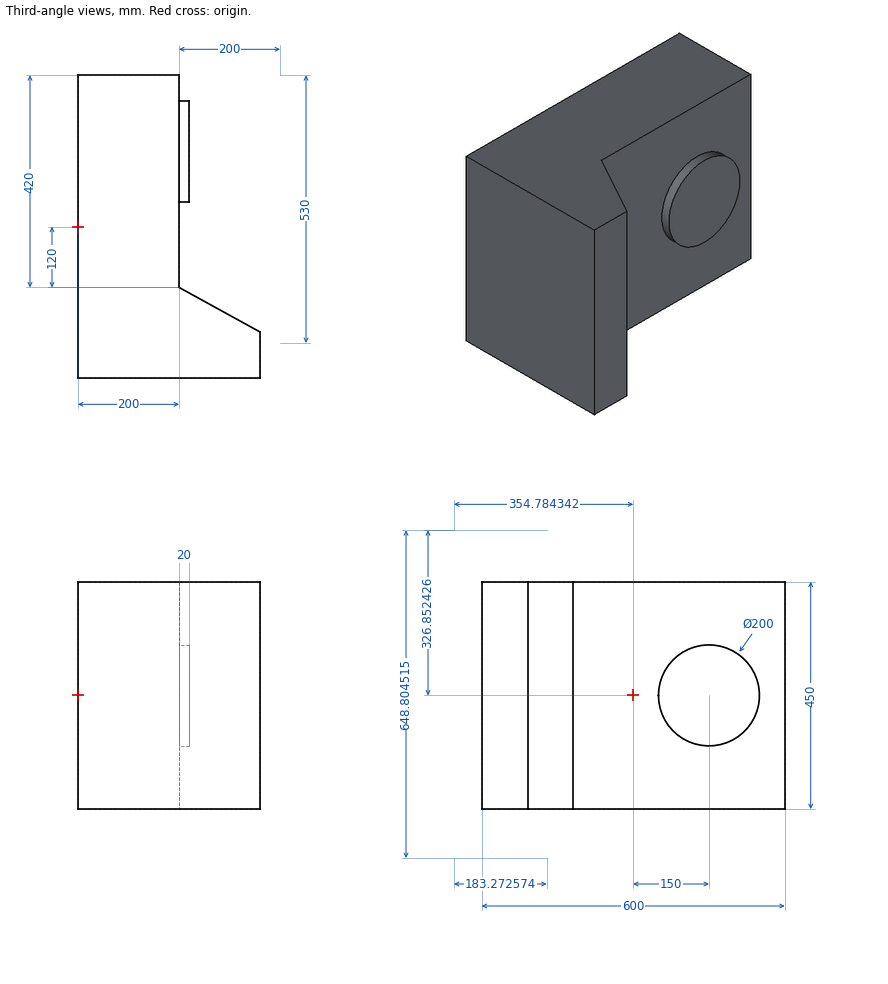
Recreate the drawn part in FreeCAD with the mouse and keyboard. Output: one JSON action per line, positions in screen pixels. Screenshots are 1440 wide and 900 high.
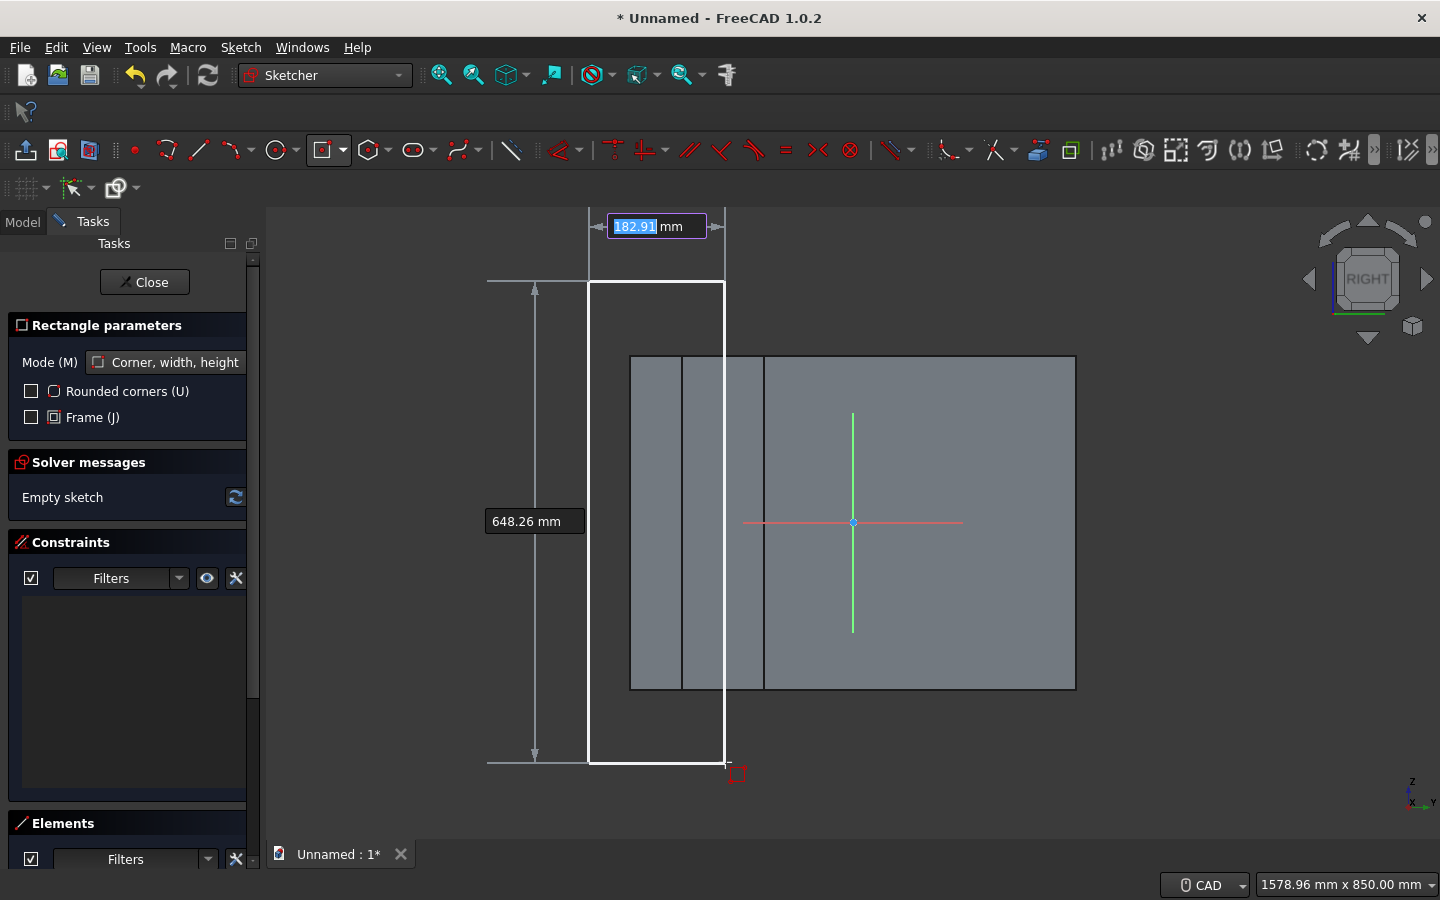
{"action": "type", "text": "183.272574"}
{"action": "key", "text": "Tab"}
{"action": "type", "text": "648.804515"}
{"action": "key", "text": "Return"}
{"action": "key", "text": "Escape"}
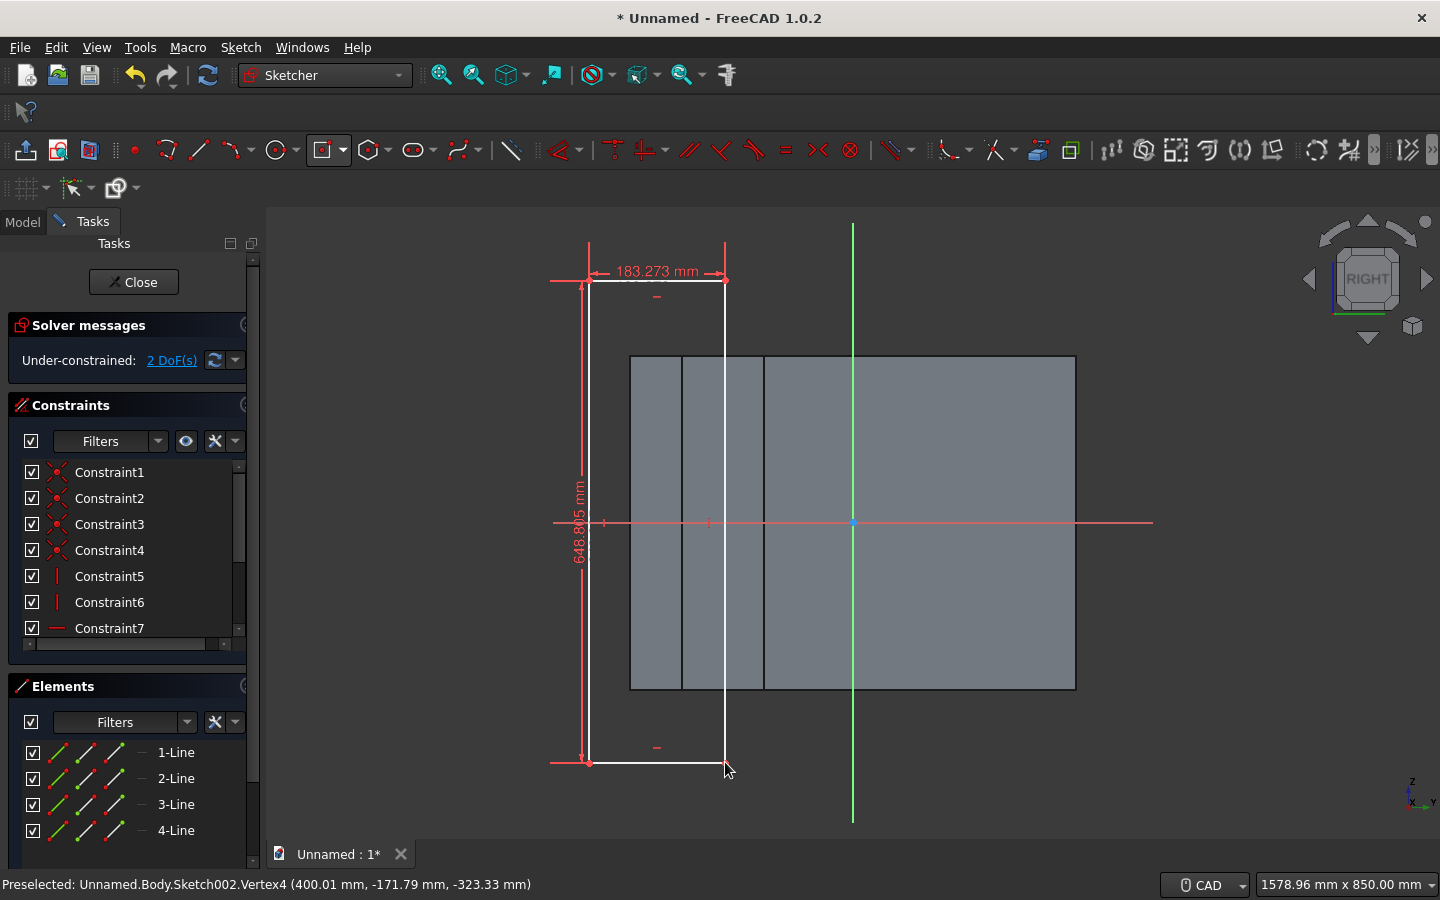
{"action": "key", "text": "d"}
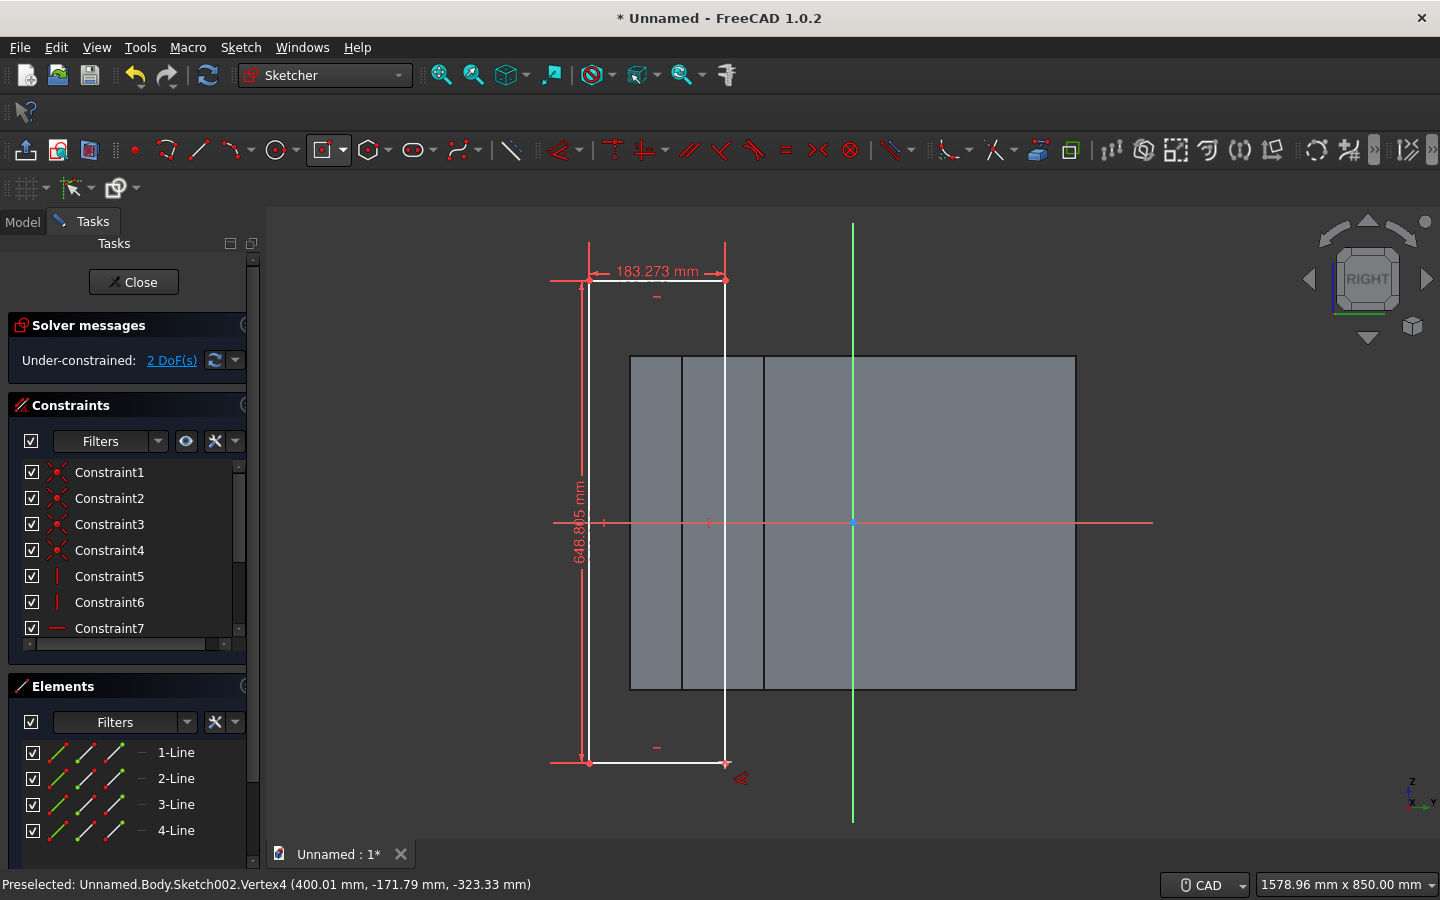
{"action": "left_click", "coordinate": [589, 281]}
{"action": "left_click", "coordinate": [721, 247]}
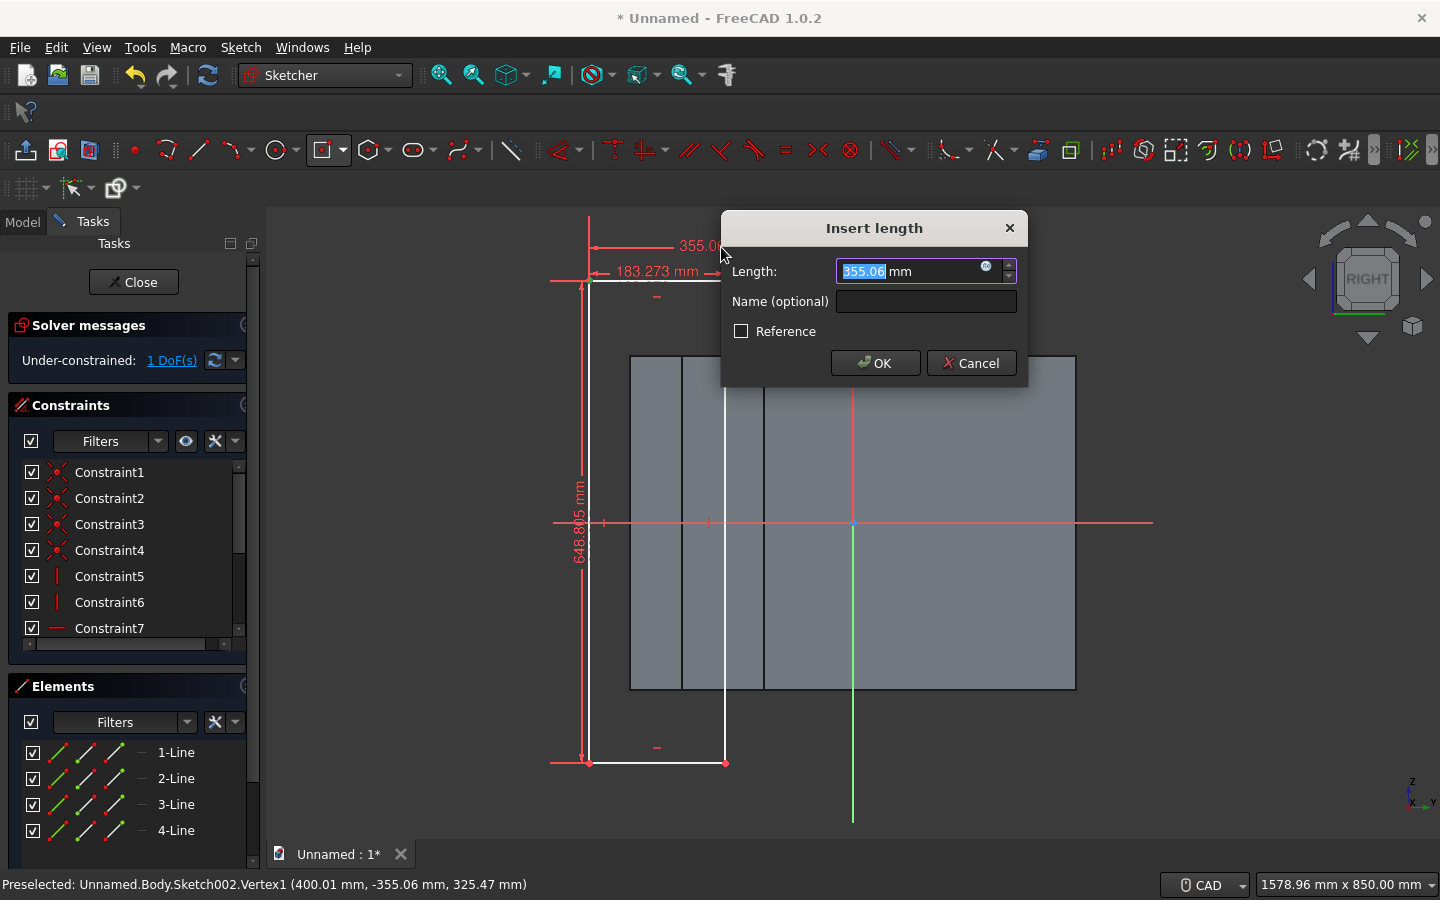
{"action": "type", "text": "354.784342"}
{"action": "key", "text": "Return"}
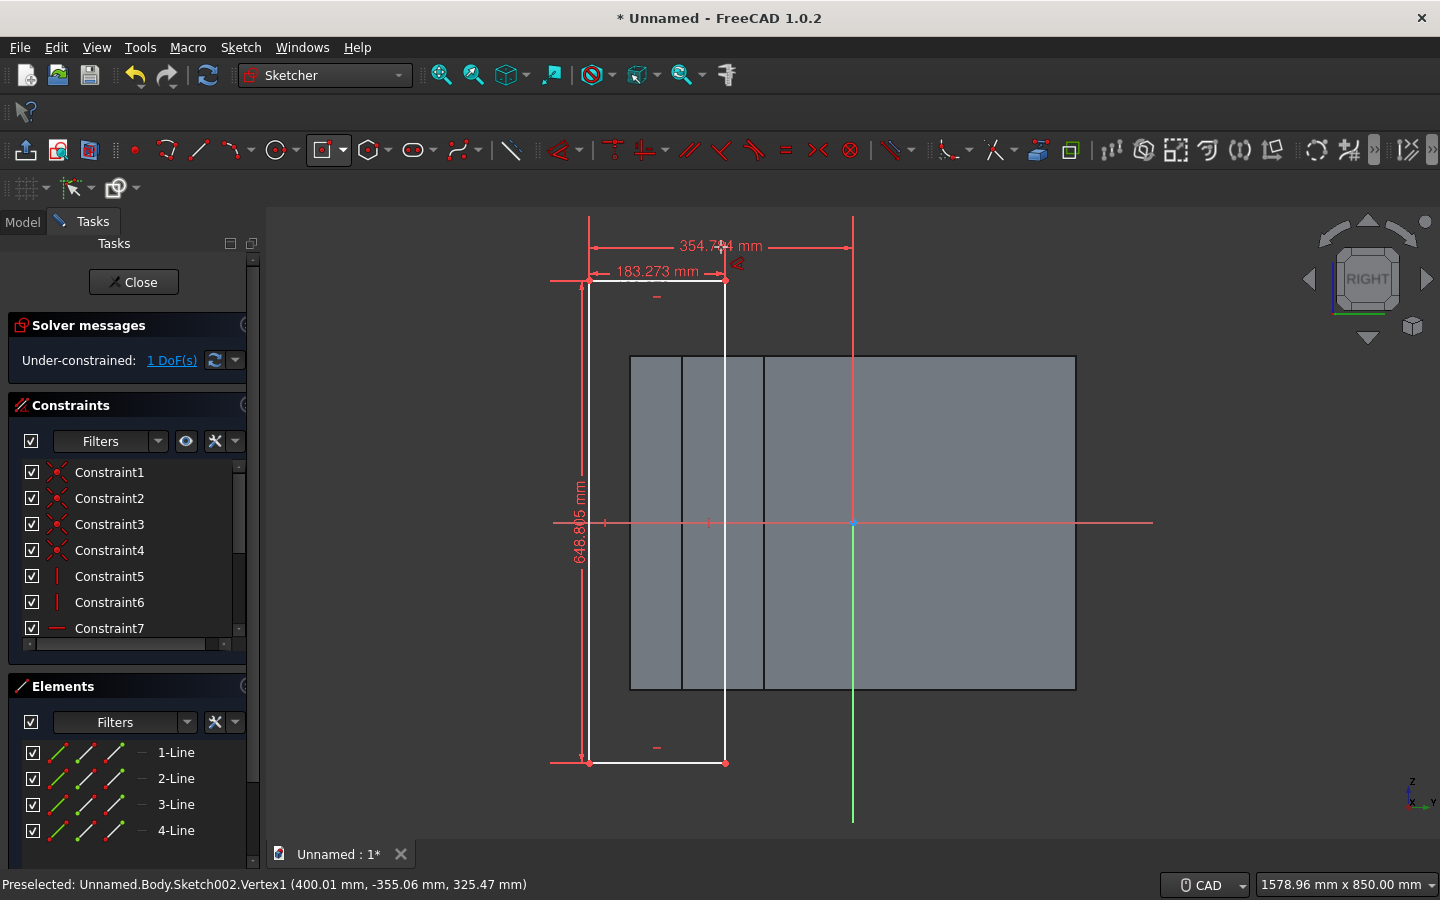
{"action": "left_click", "coordinate": [589, 281]}
{"action": "left_click", "coordinate": [555, 402]}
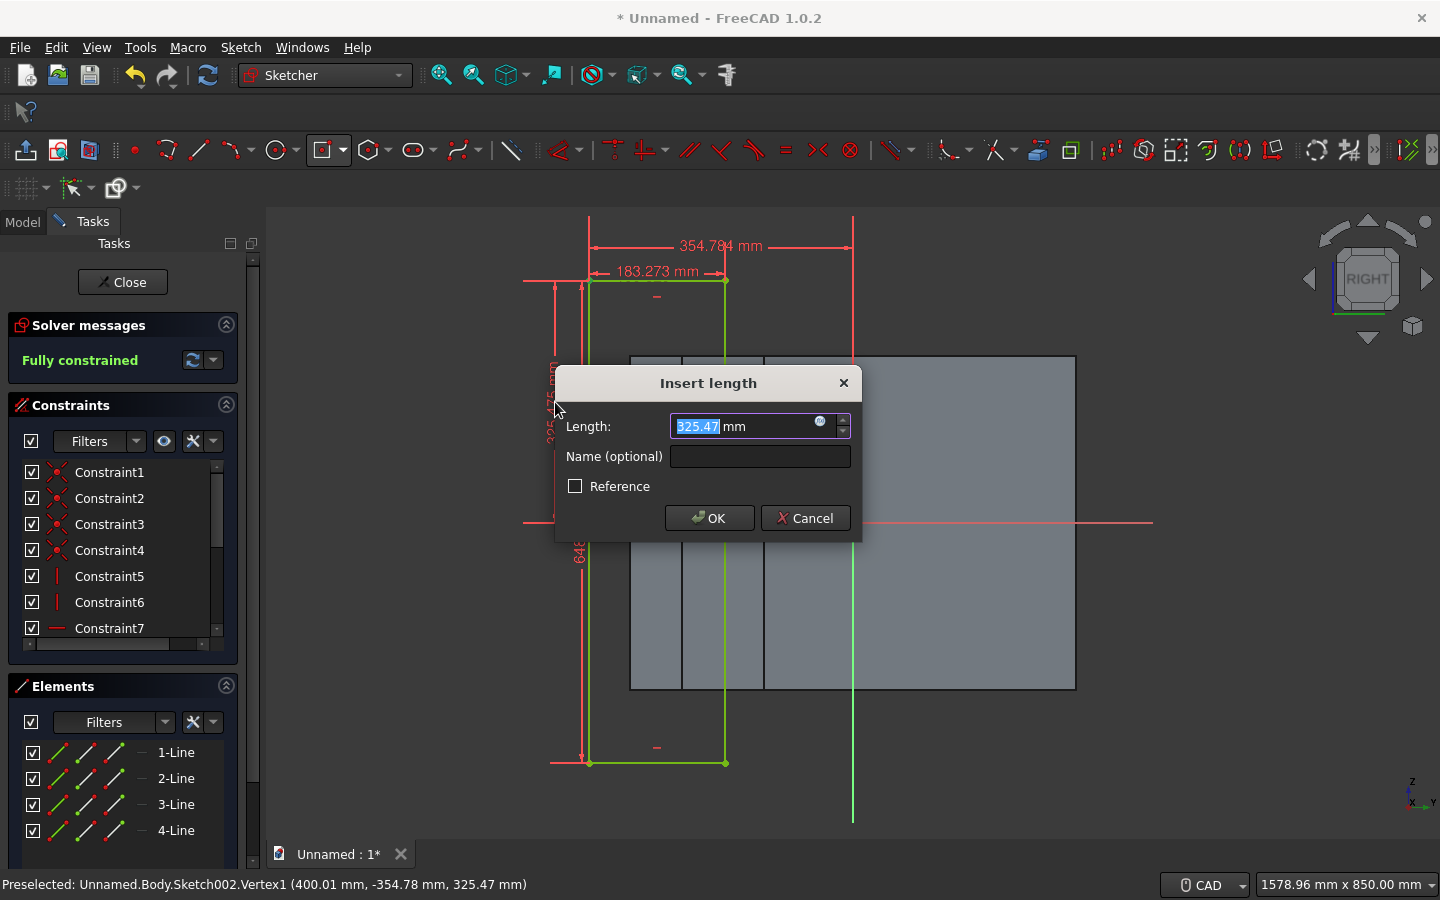
{"action": "type", "text": "326.852426"}
{"action": "key", "text": "Return"}
{"action": "key", "text": "Escape"}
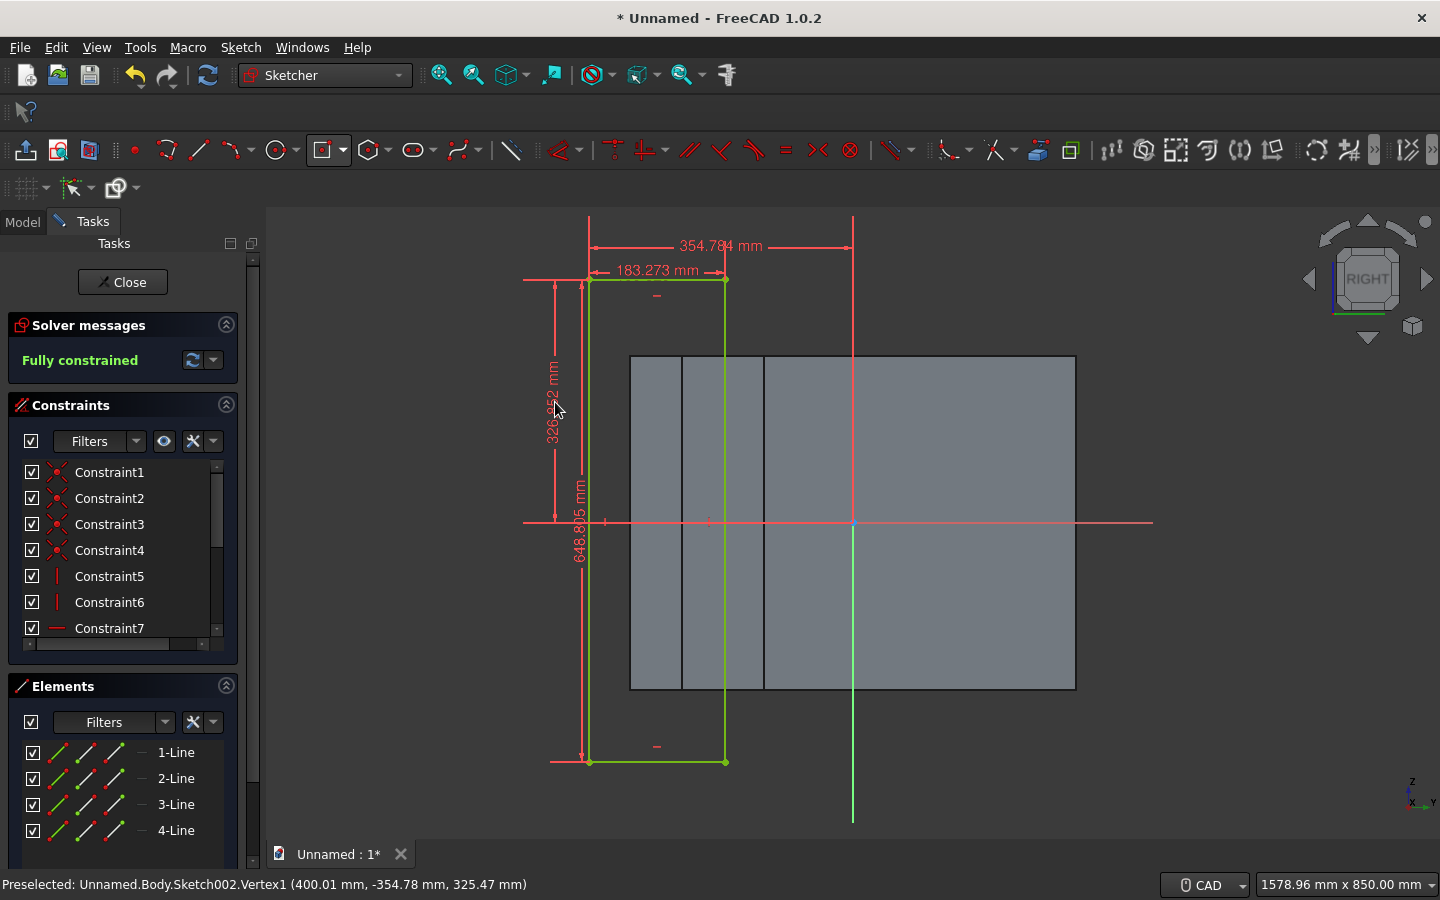
{"action": "left_click", "coordinate": [123, 282]}